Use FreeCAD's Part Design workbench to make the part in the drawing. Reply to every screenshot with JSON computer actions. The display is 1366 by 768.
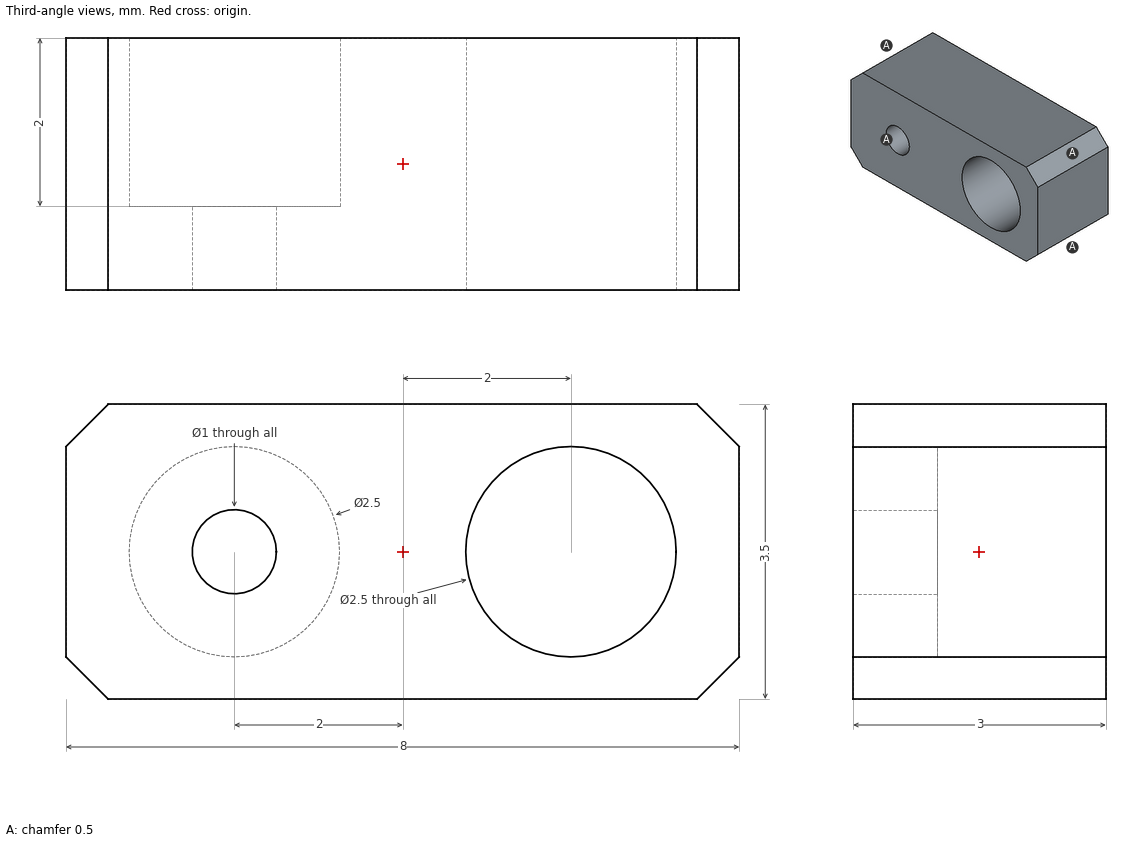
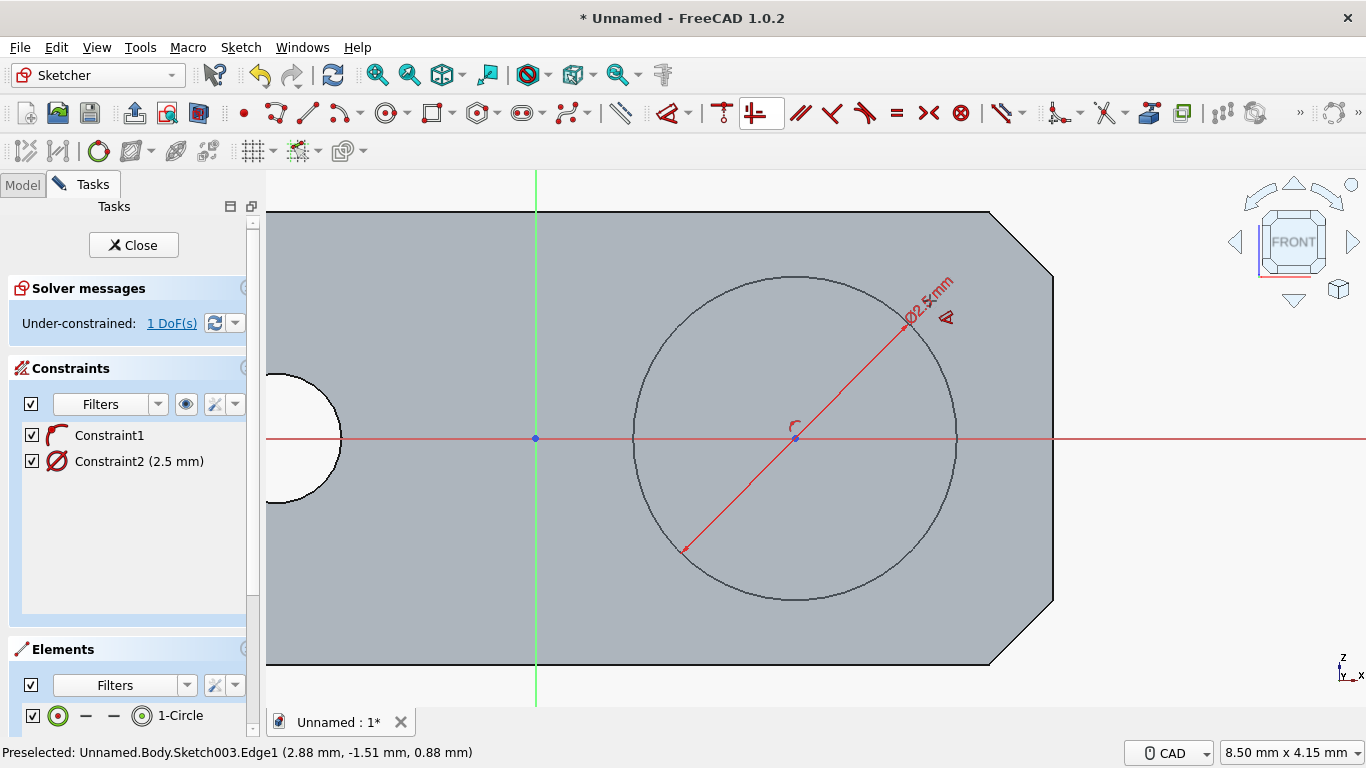
{"action": "left_click", "coordinate": [795, 438]}
{"action": "left_click", "coordinate": [665, 472]}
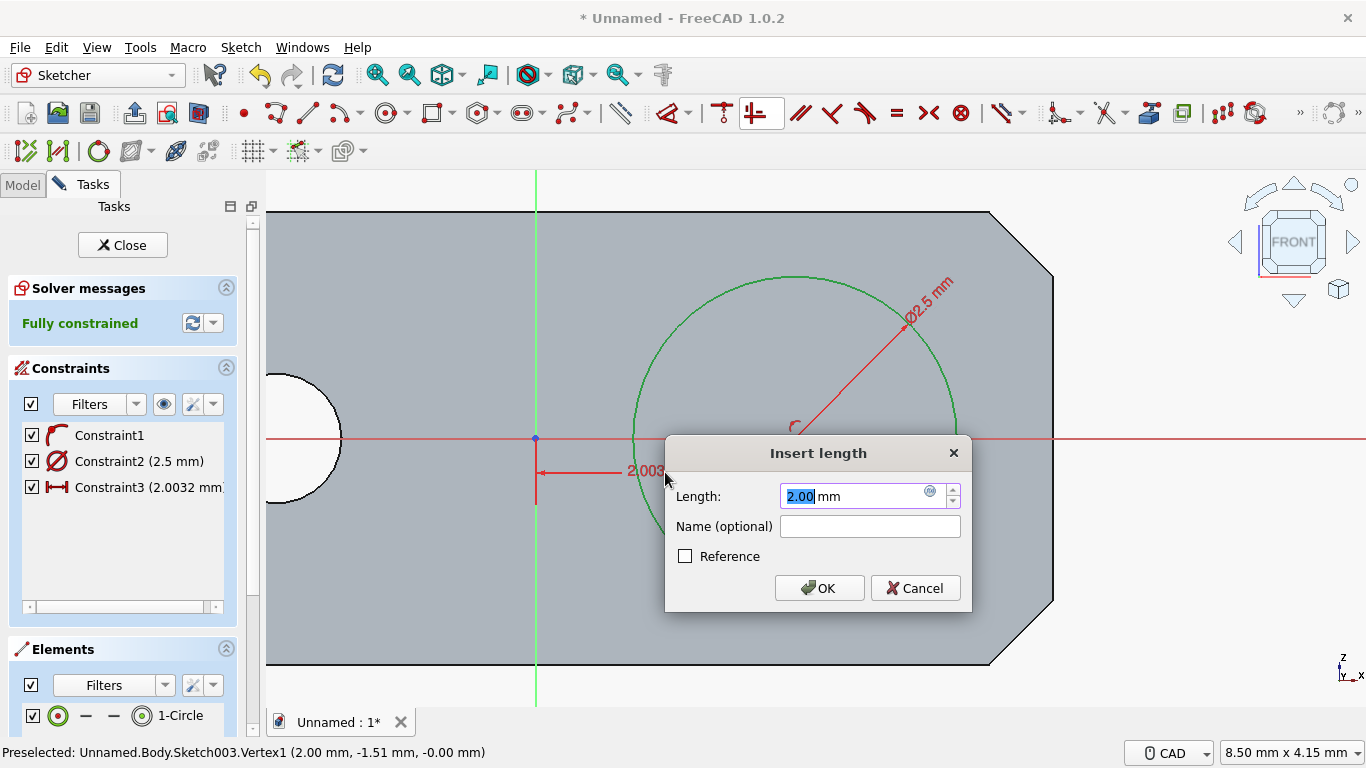
{"action": "type", "text": "2"}
{"action": "key", "text": "Return"}
{"action": "key", "text": "Escape"}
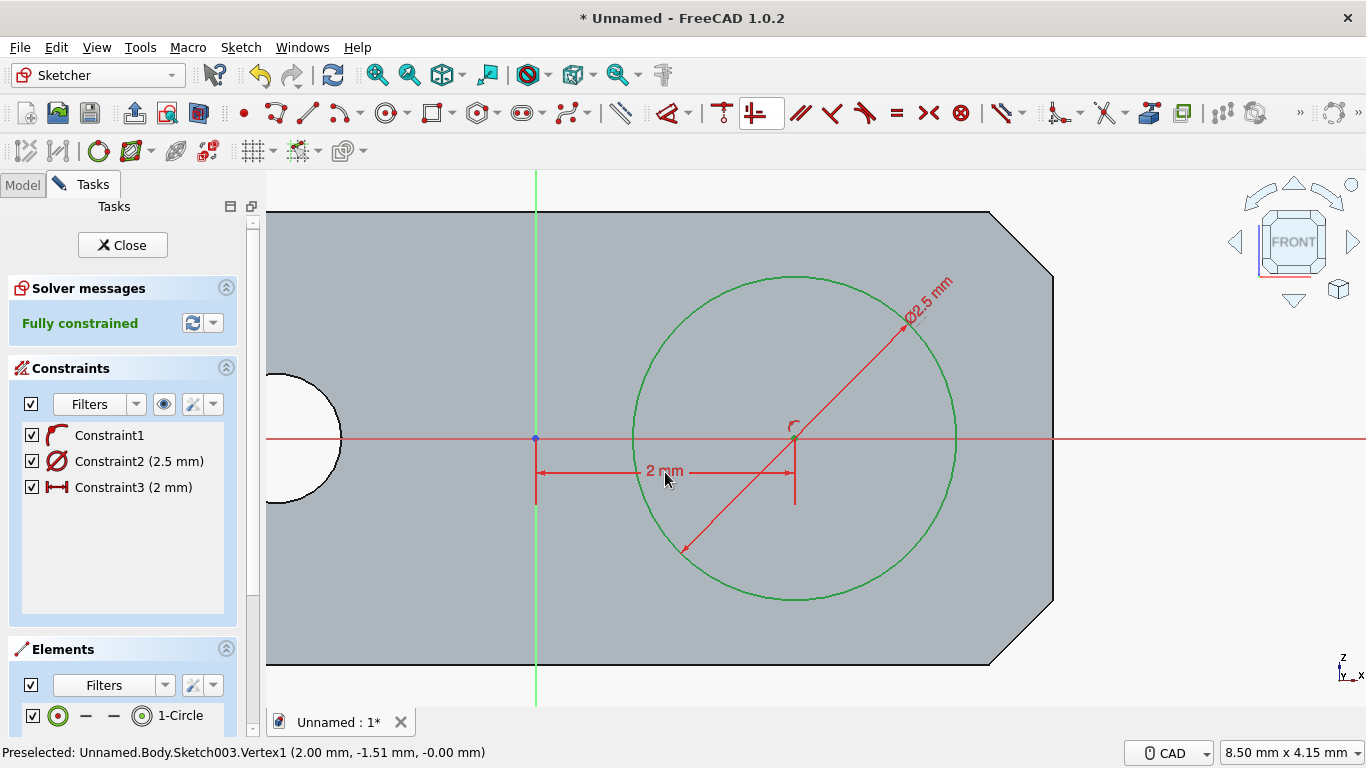
{"action": "left_click", "coordinate": [123, 245]}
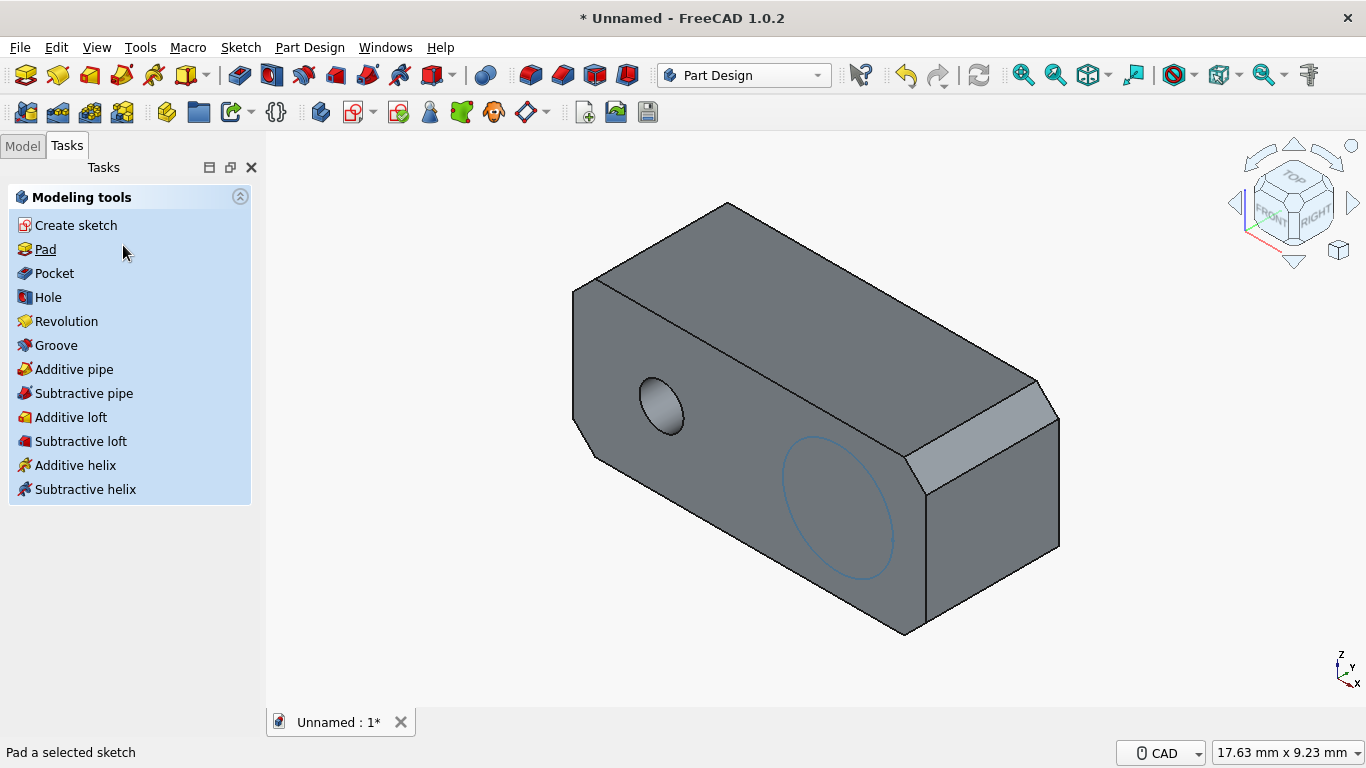
{"action": "left_click", "coordinate": [272, 76]}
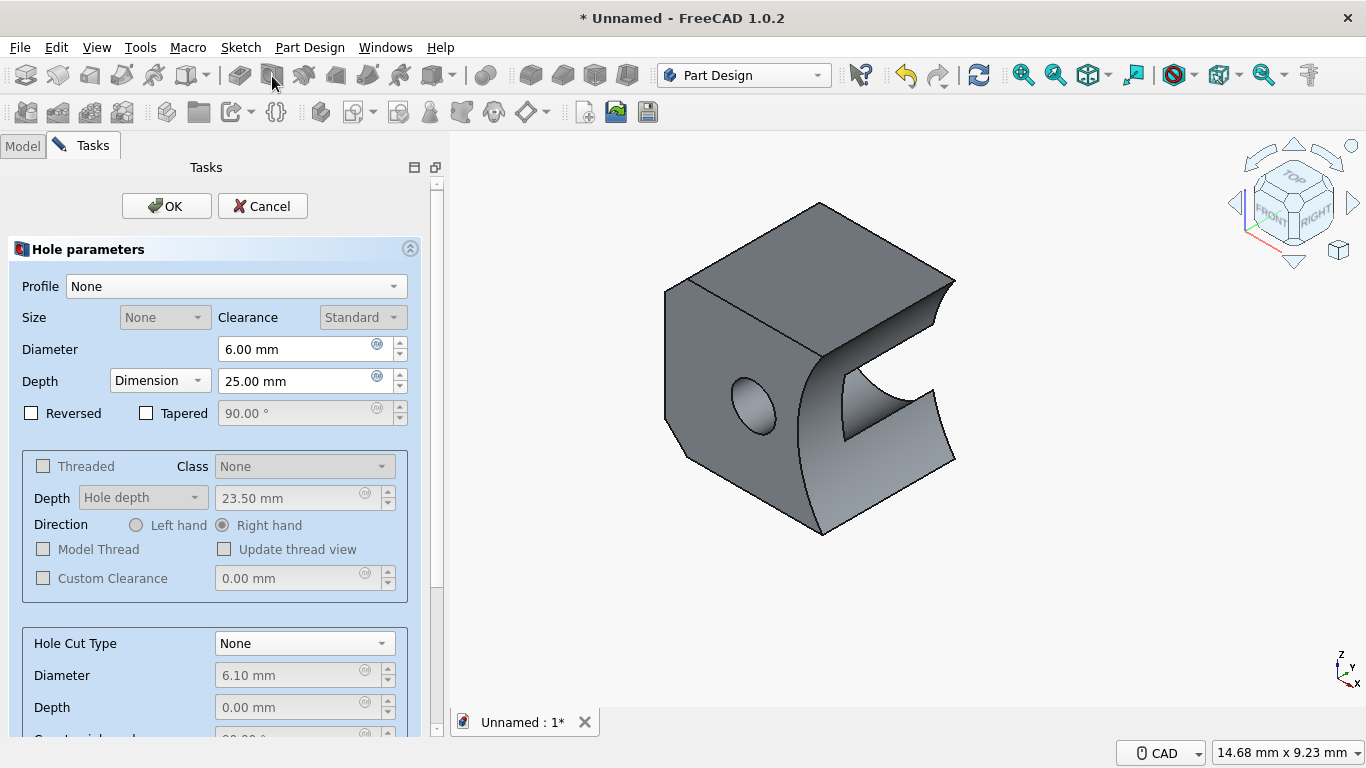
{"action": "triple_click", "coordinate": [305, 349]}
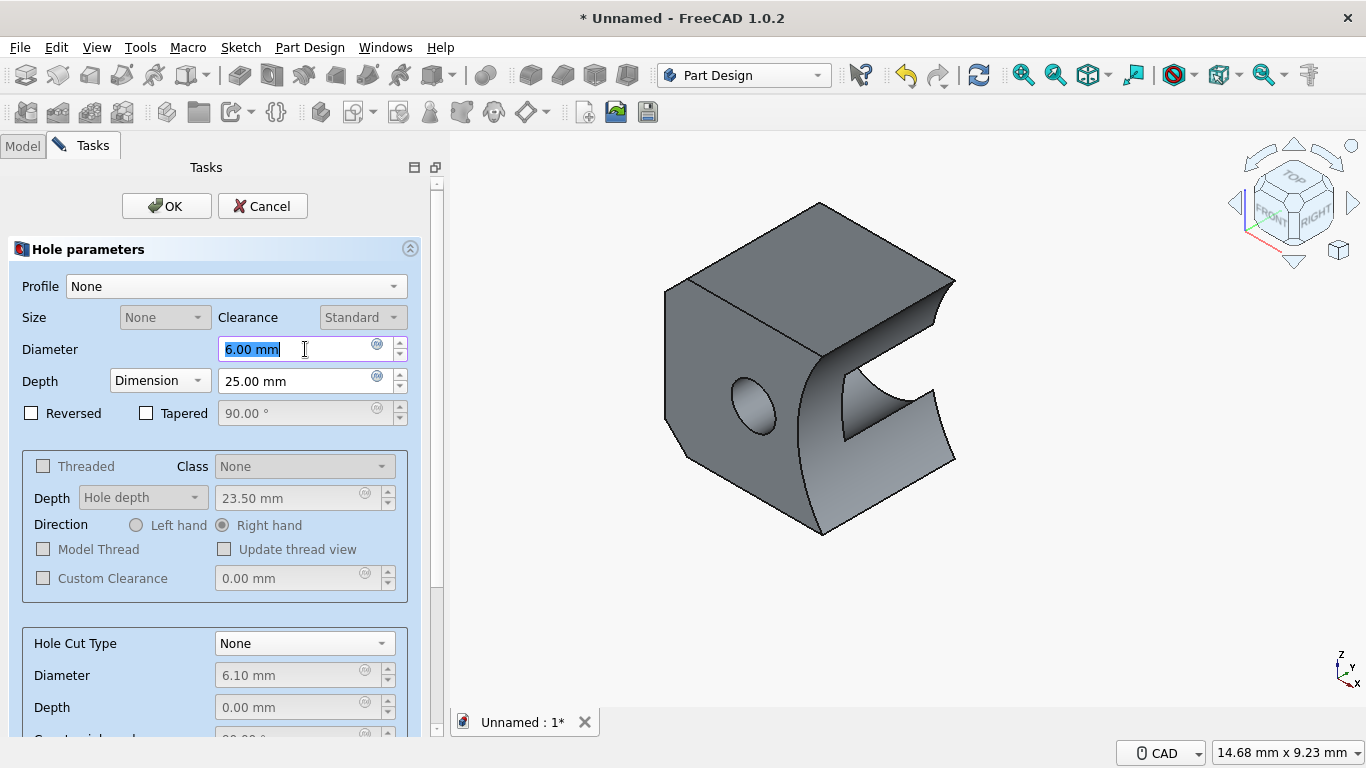
{"action": "type", "text": "2.5"}
{"action": "key", "text": "Tab"}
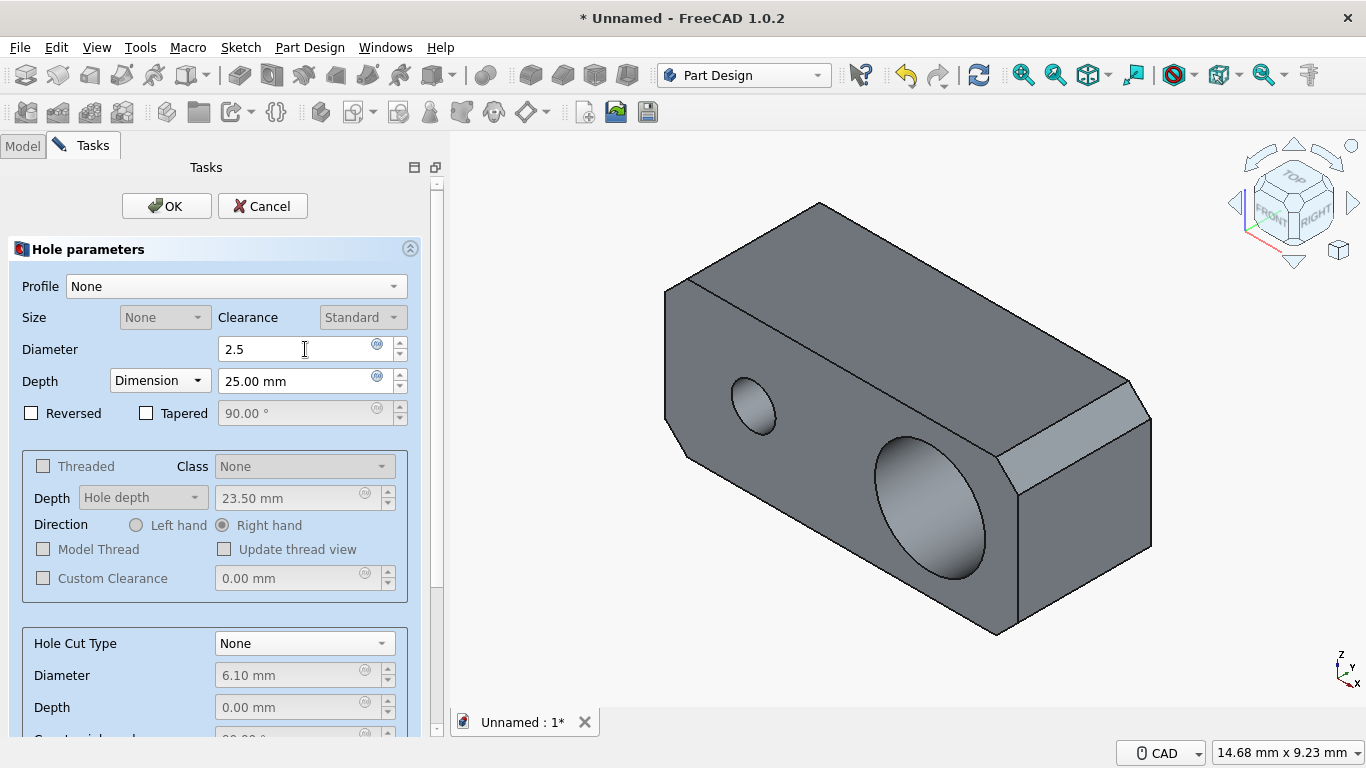
{"action": "left_click", "coordinate": [161, 380]}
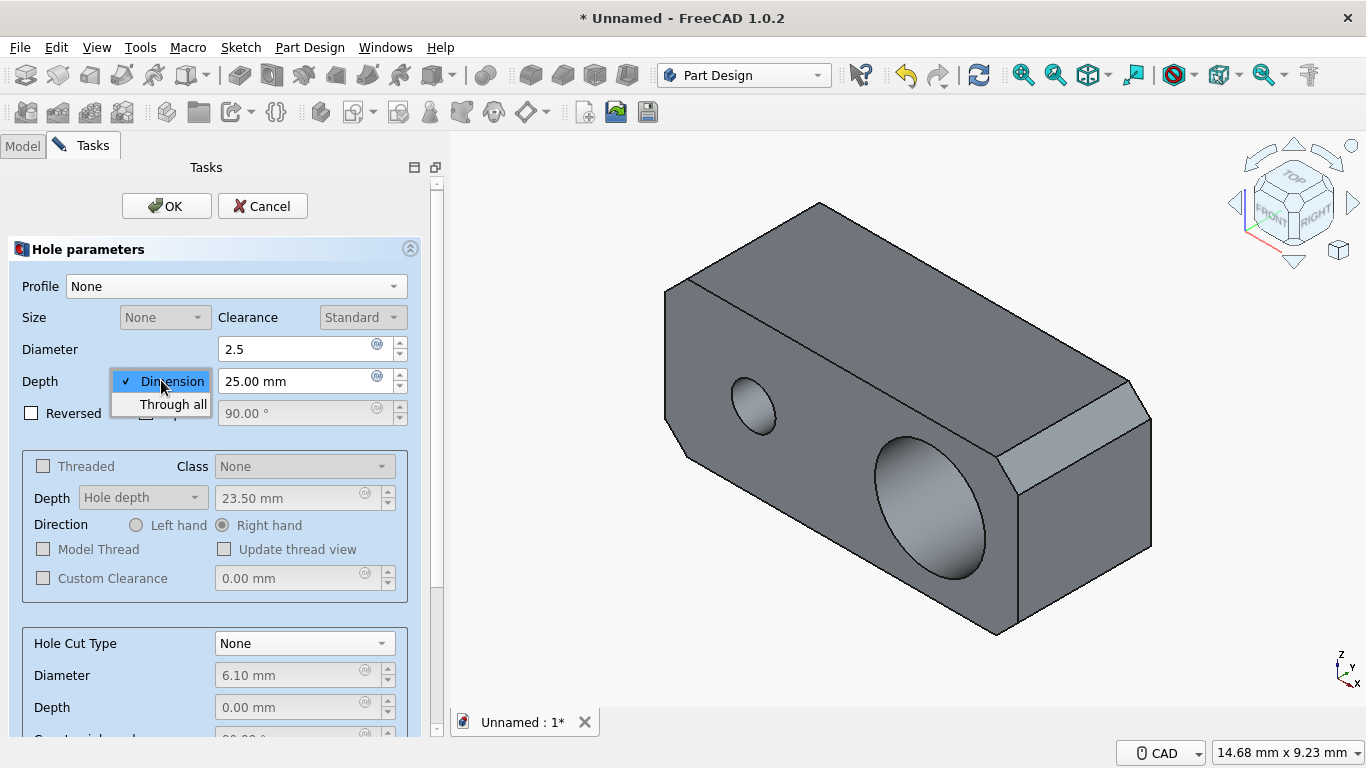
{"action": "left_click", "coordinate": [160, 404]}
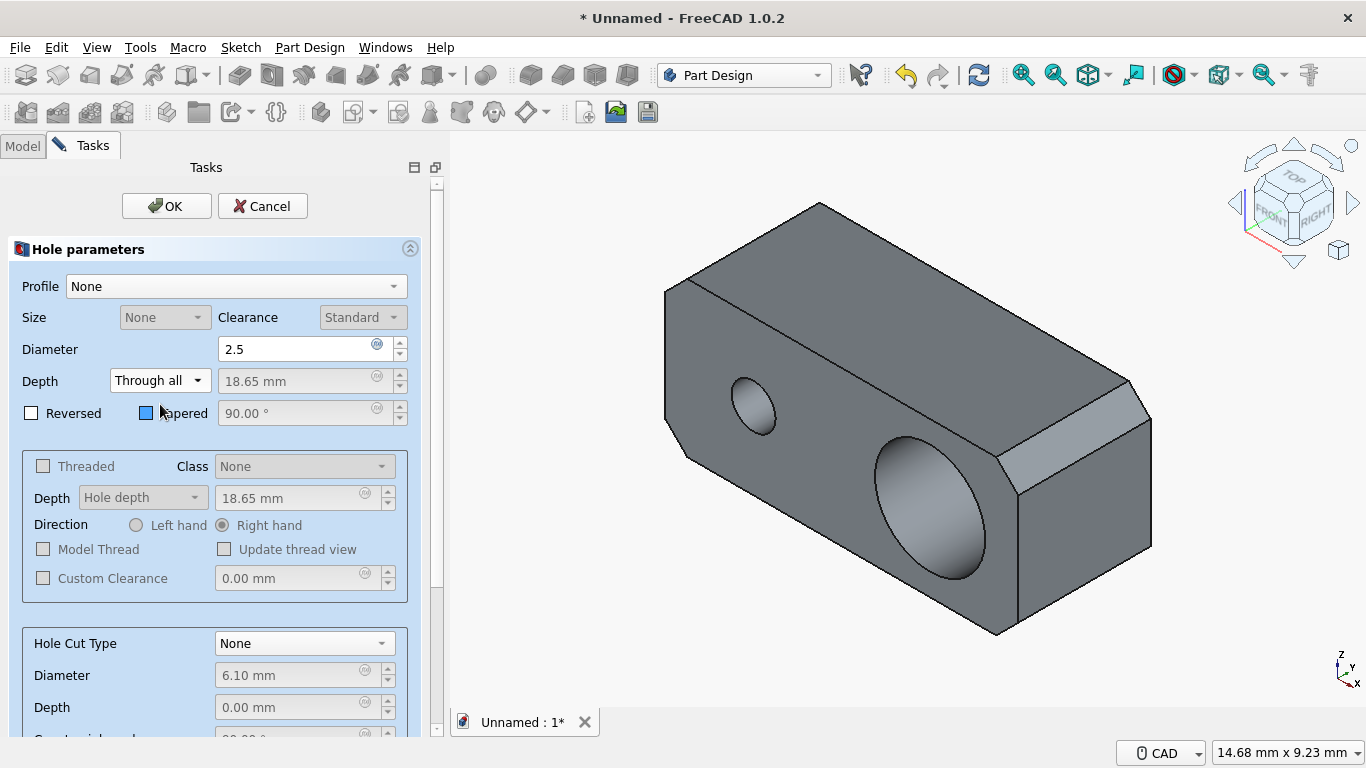
{"action": "left_click", "coordinate": [167, 206]}